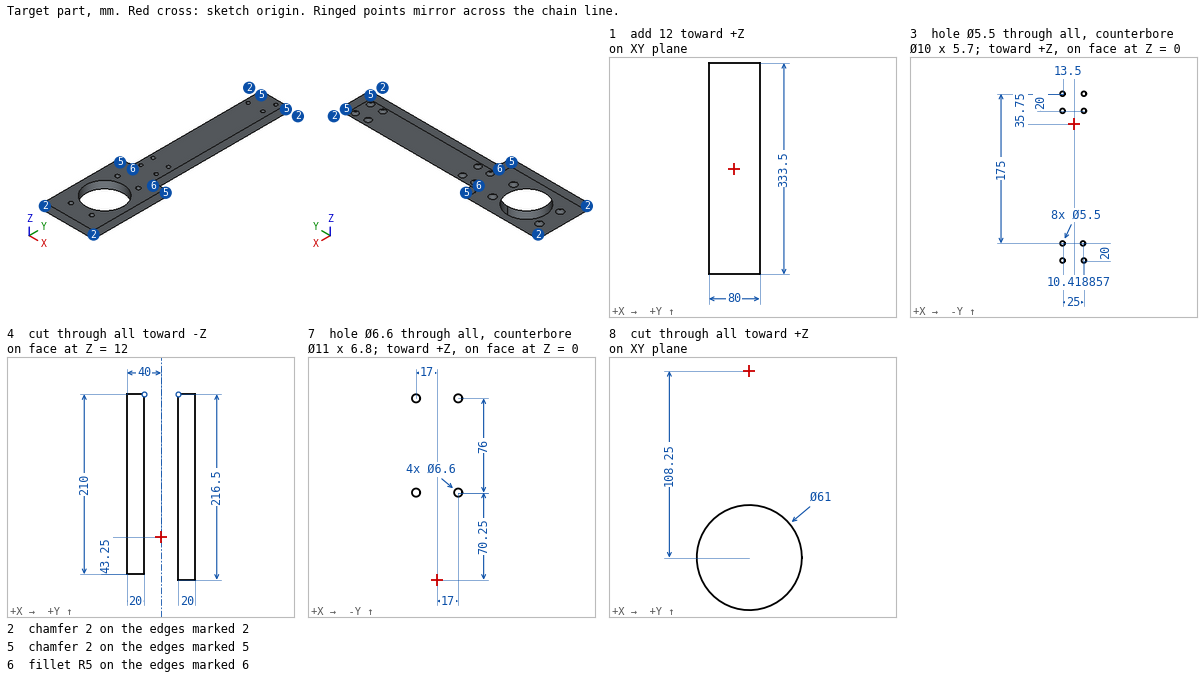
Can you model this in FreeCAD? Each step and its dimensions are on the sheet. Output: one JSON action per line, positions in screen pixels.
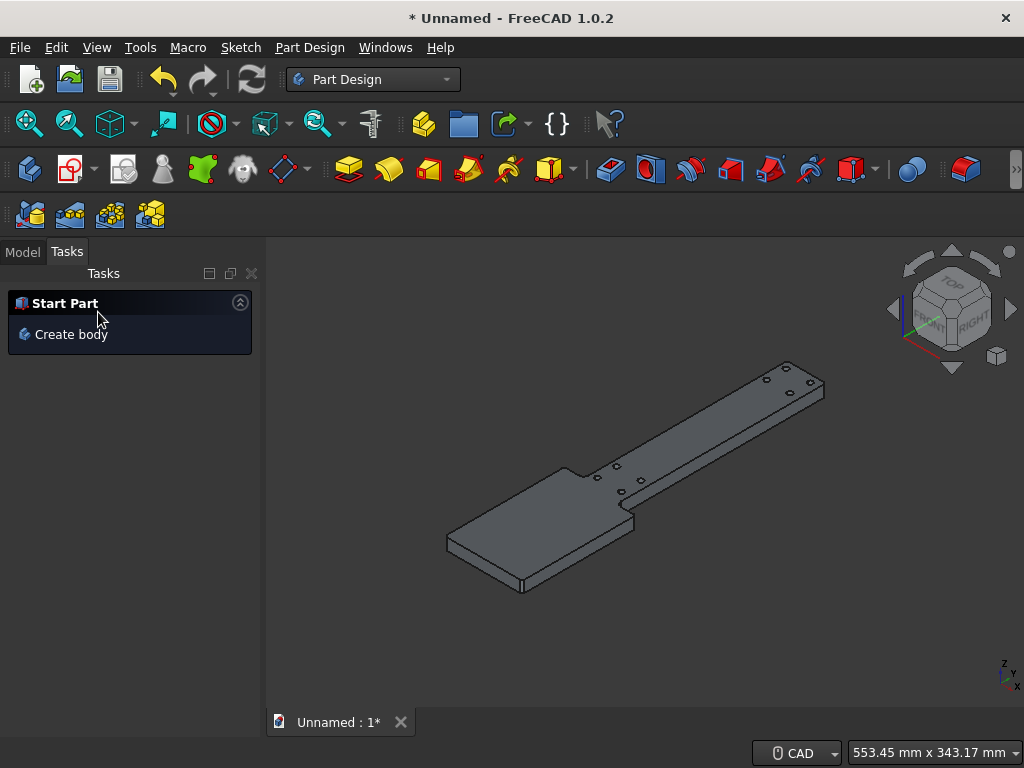
{"action": "key", "text": "5"}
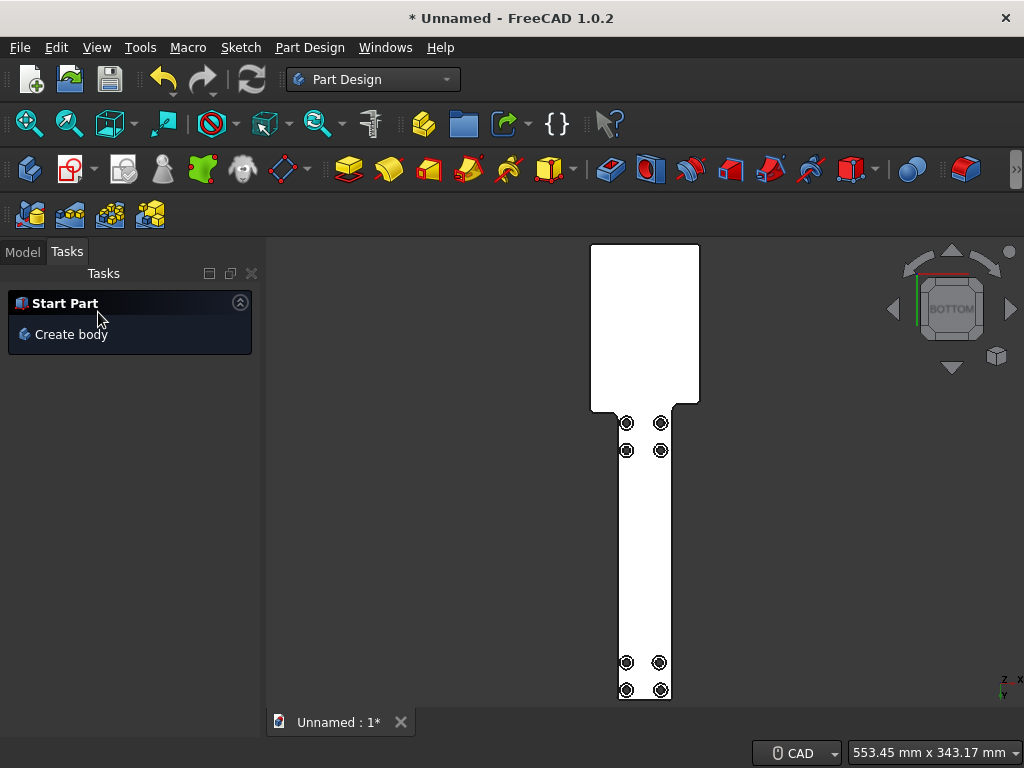
{"action": "left_click", "coordinate": [645, 340]}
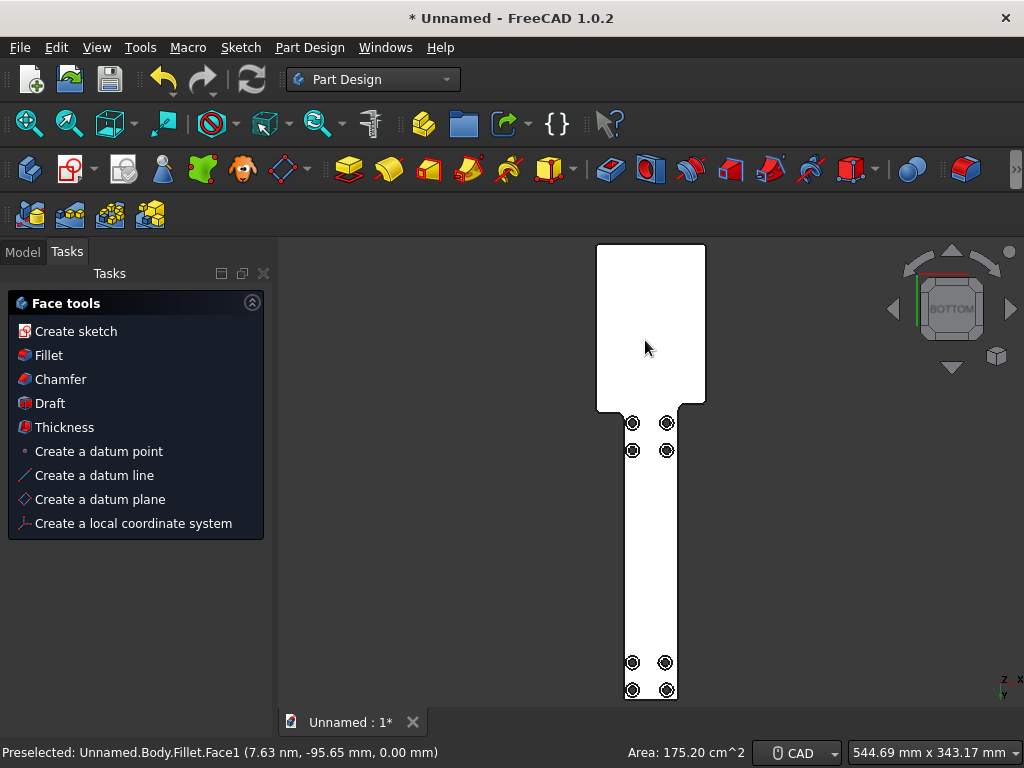
{"action": "left_click", "coordinate": [70, 170]}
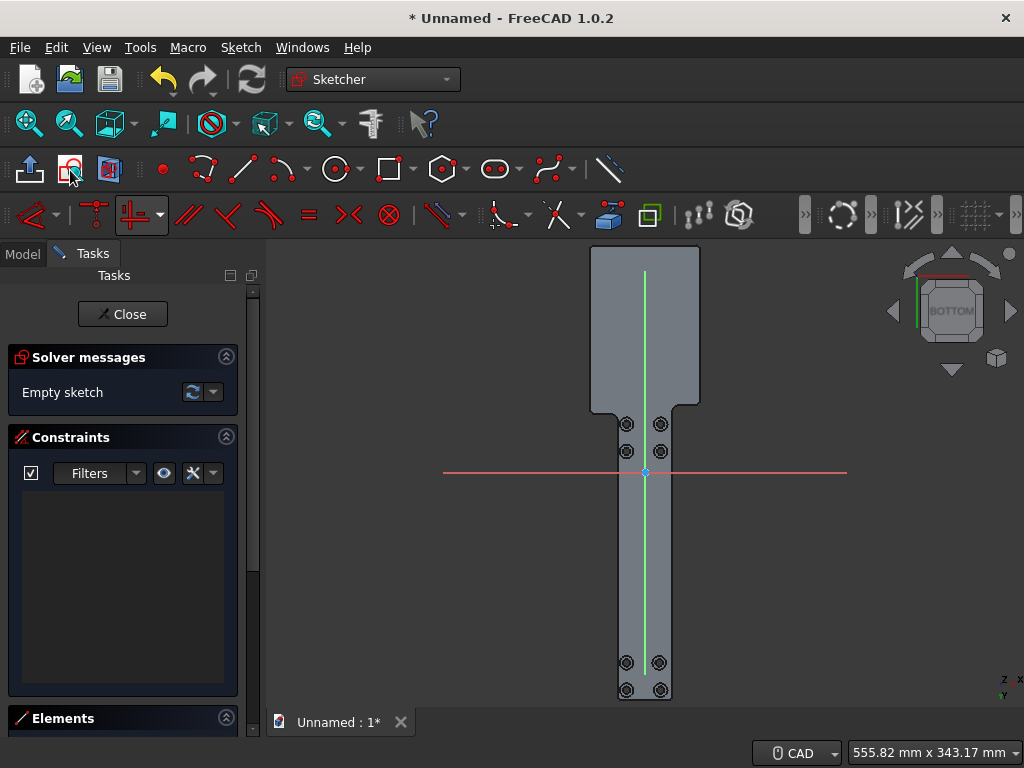
{"action": "scroll", "coordinate": [294, 679], "scroll_direction": "down", "scroll_amount": 1}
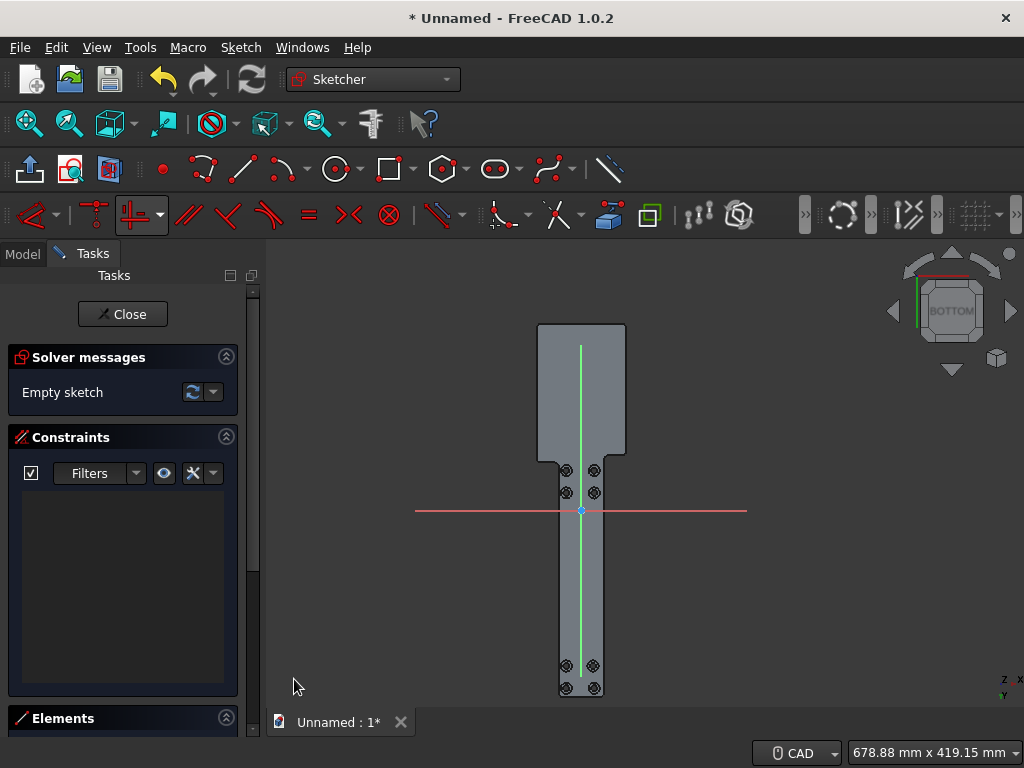
{"action": "scroll", "coordinate": [587, 371], "scroll_direction": "up", "scroll_amount": 3}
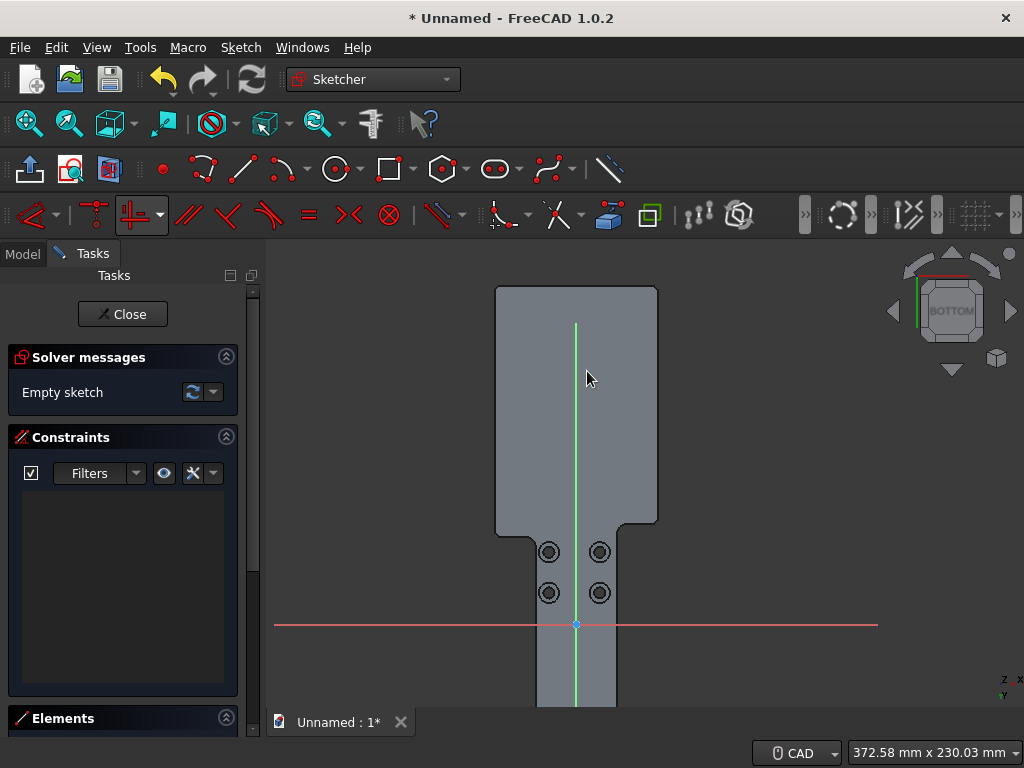
{"action": "left_click", "coordinate": [336, 170]}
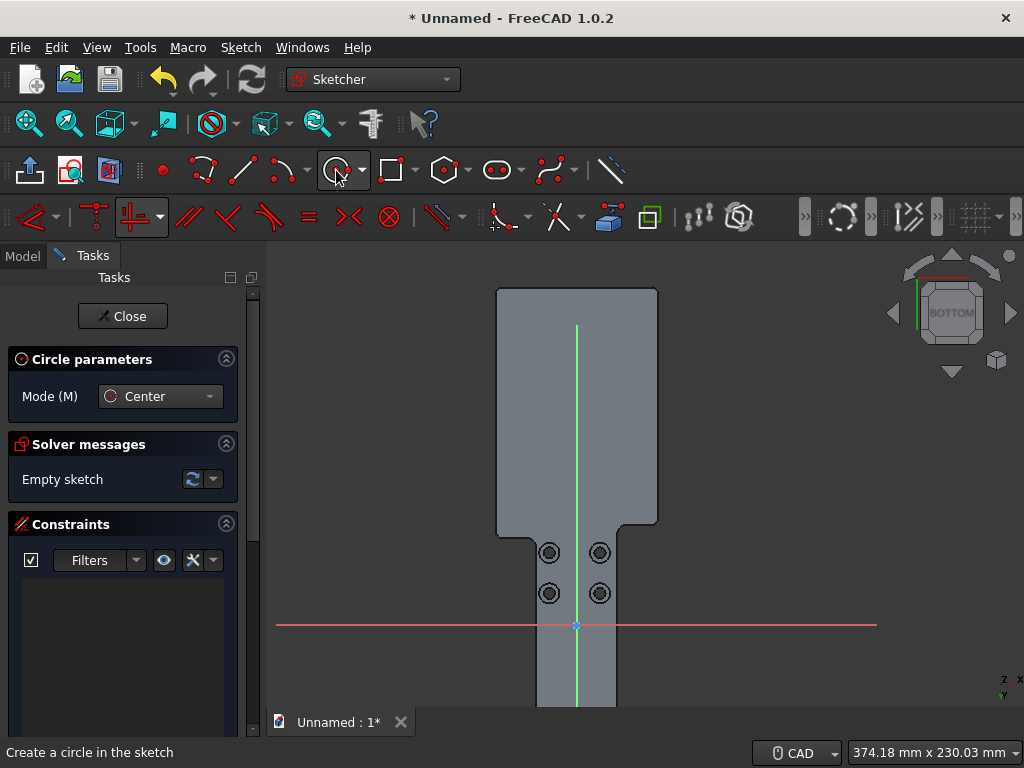
{"action": "scroll", "coordinate": [611, 483], "scroll_direction": "up", "scroll_amount": 7}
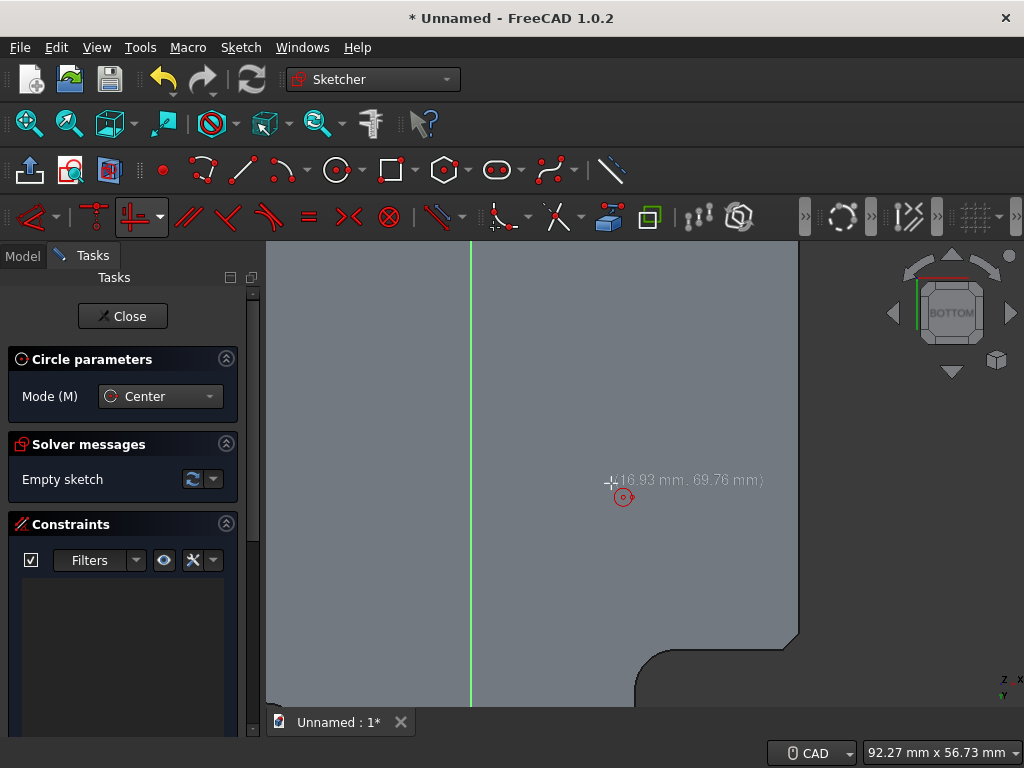
{"action": "scroll", "coordinate": [611, 484], "scroll_direction": "down", "scroll_amount": 7}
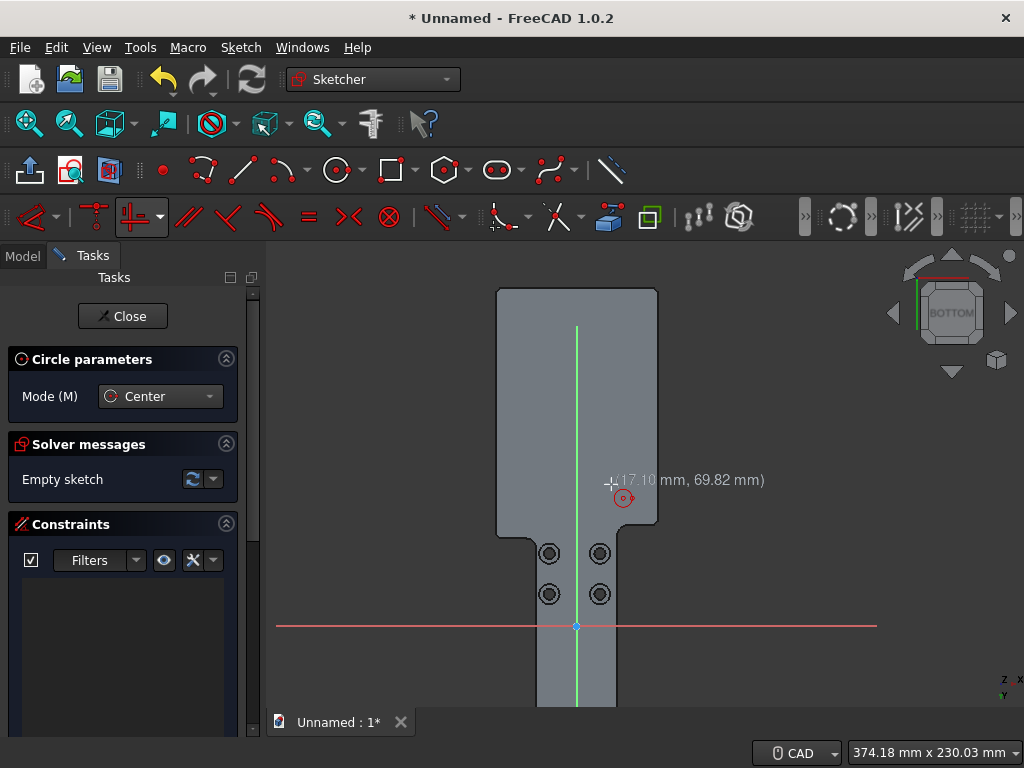
{"action": "left_click", "coordinate": [611, 484]}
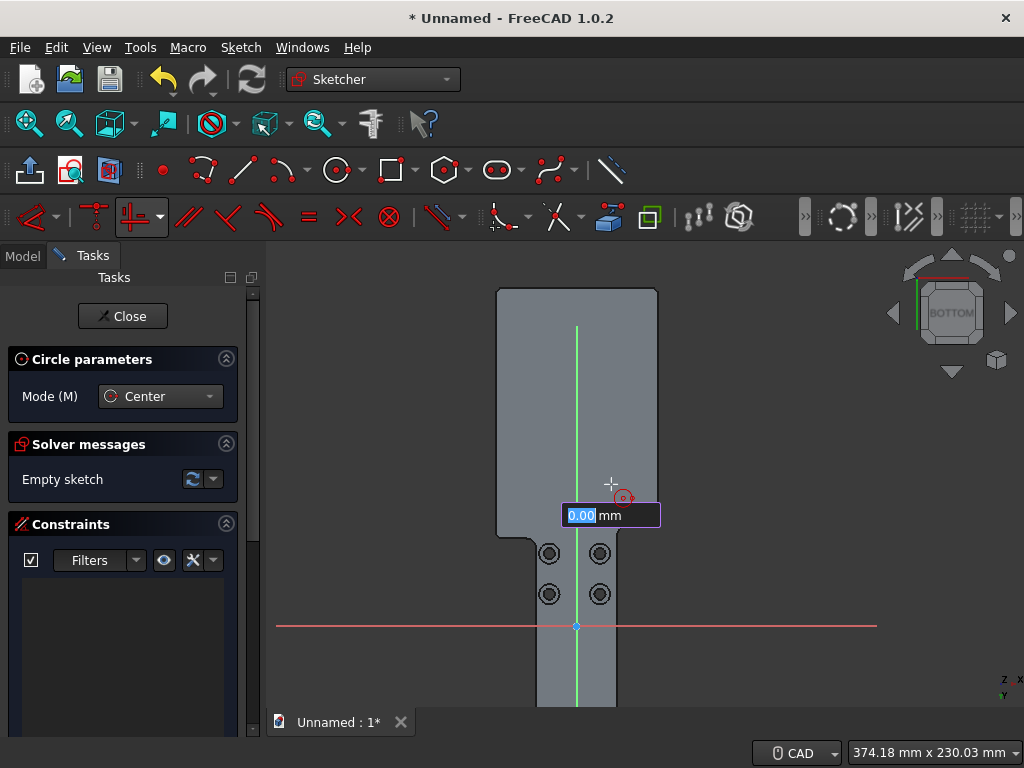
{"action": "scroll", "coordinate": [616, 479], "scroll_direction": "up", "scroll_amount": 5}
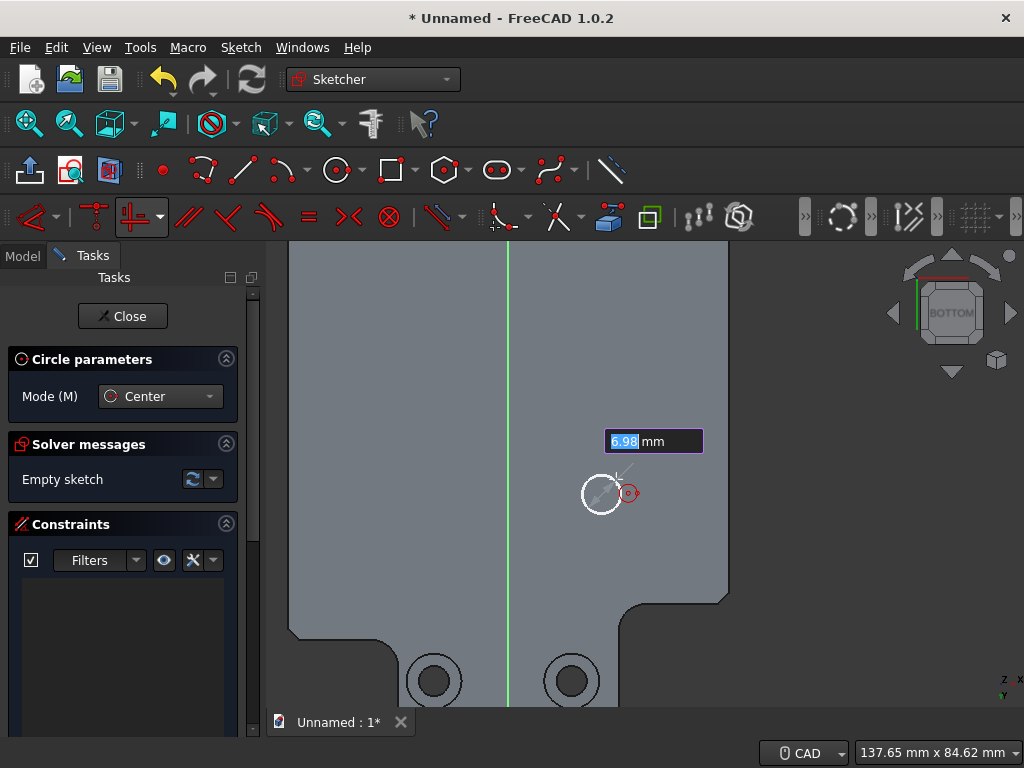
{"action": "left_click", "coordinate": [615, 478]}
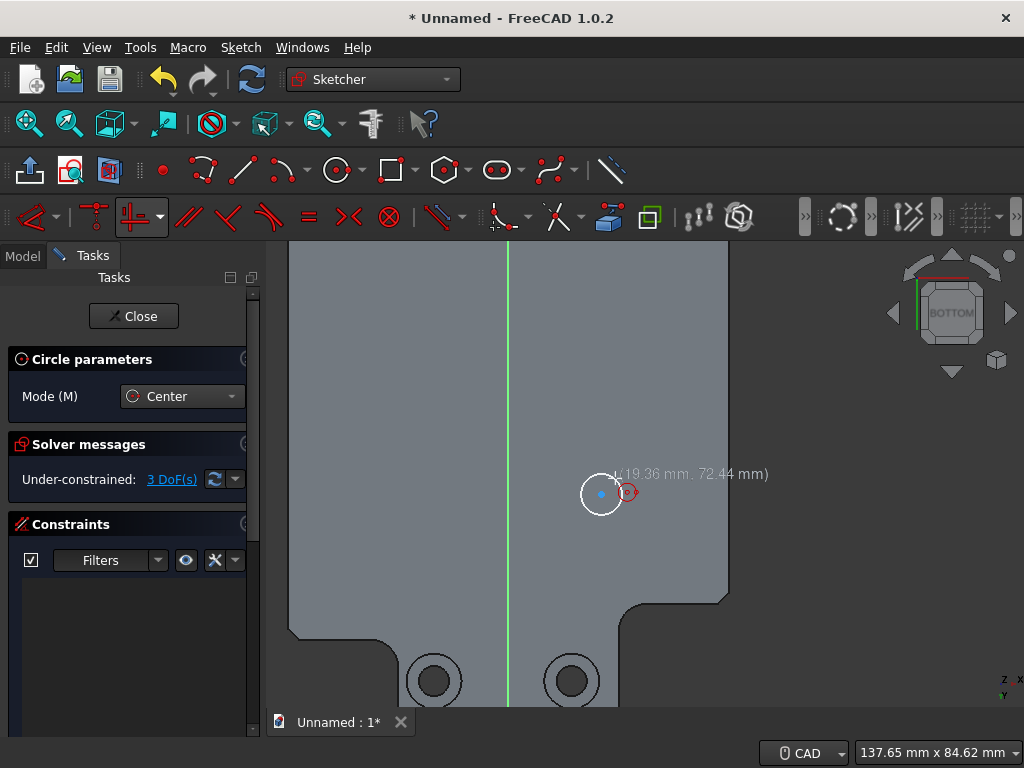
{"action": "scroll", "coordinate": [616, 479], "scroll_direction": "down", "scroll_amount": 5}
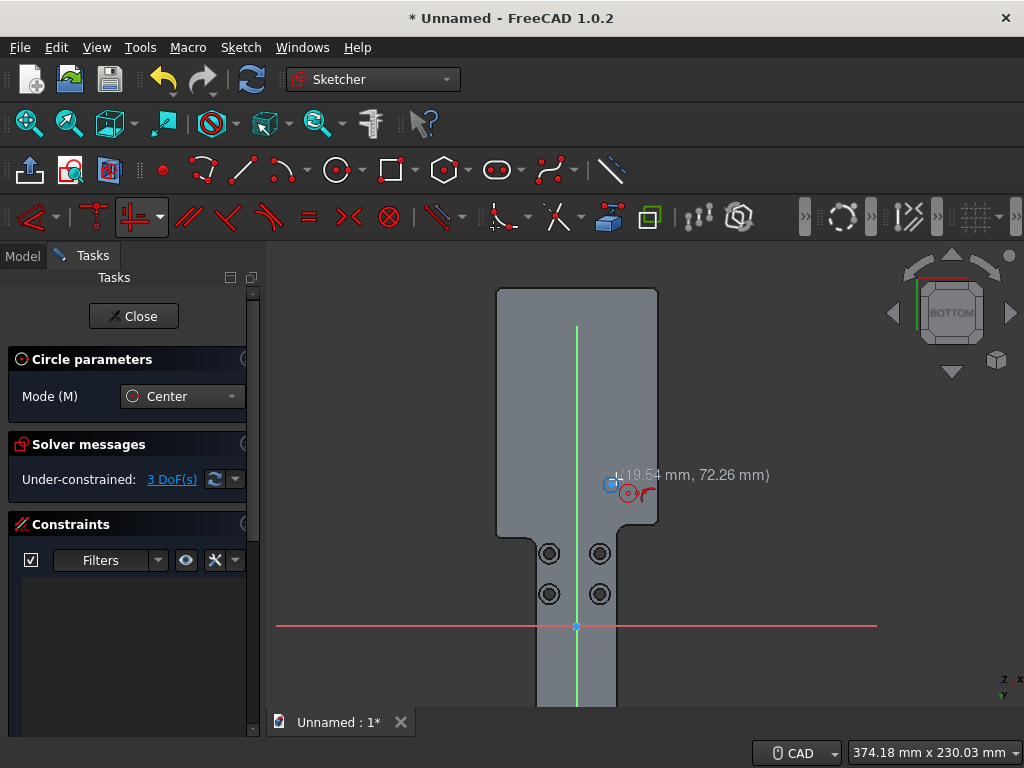
{"action": "scroll", "coordinate": [611, 330], "scroll_direction": "up", "scroll_amount": 7}